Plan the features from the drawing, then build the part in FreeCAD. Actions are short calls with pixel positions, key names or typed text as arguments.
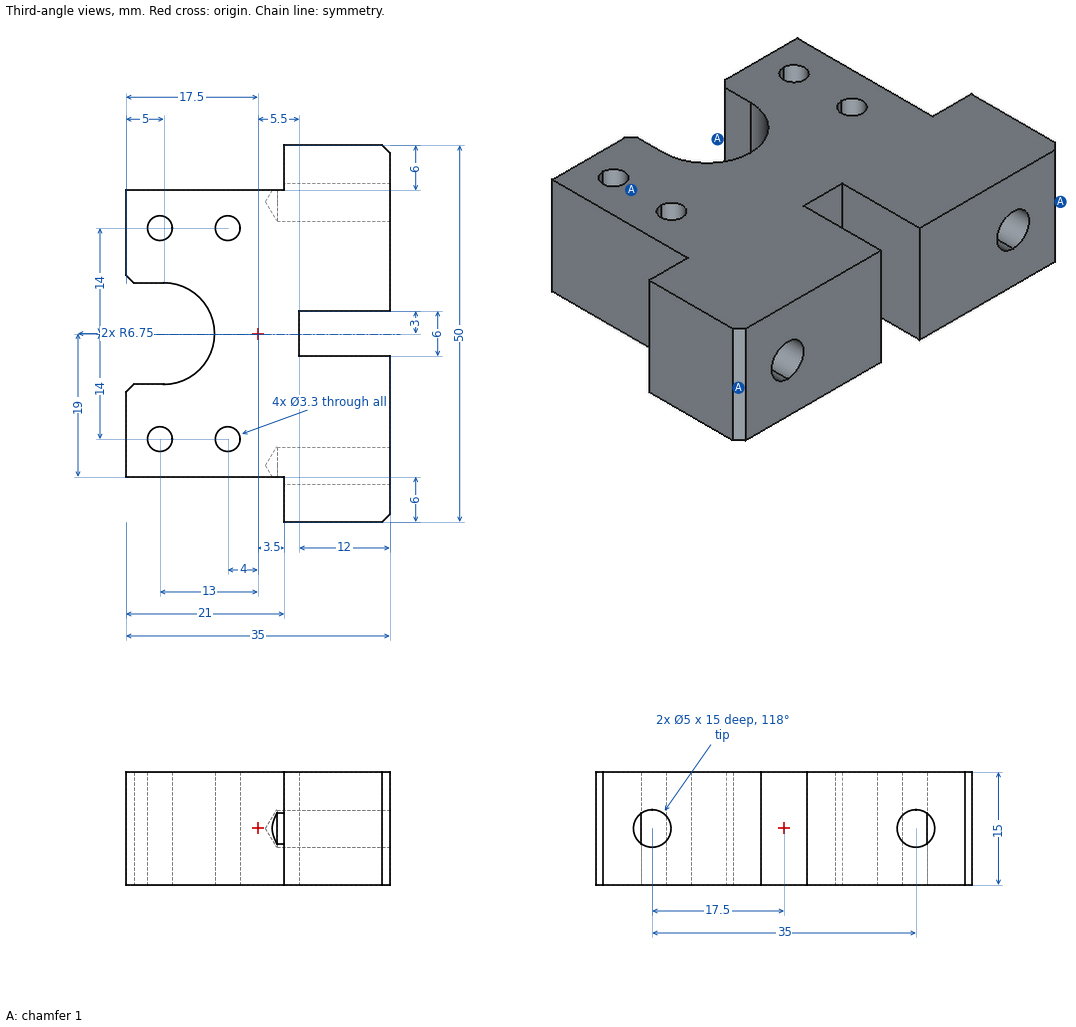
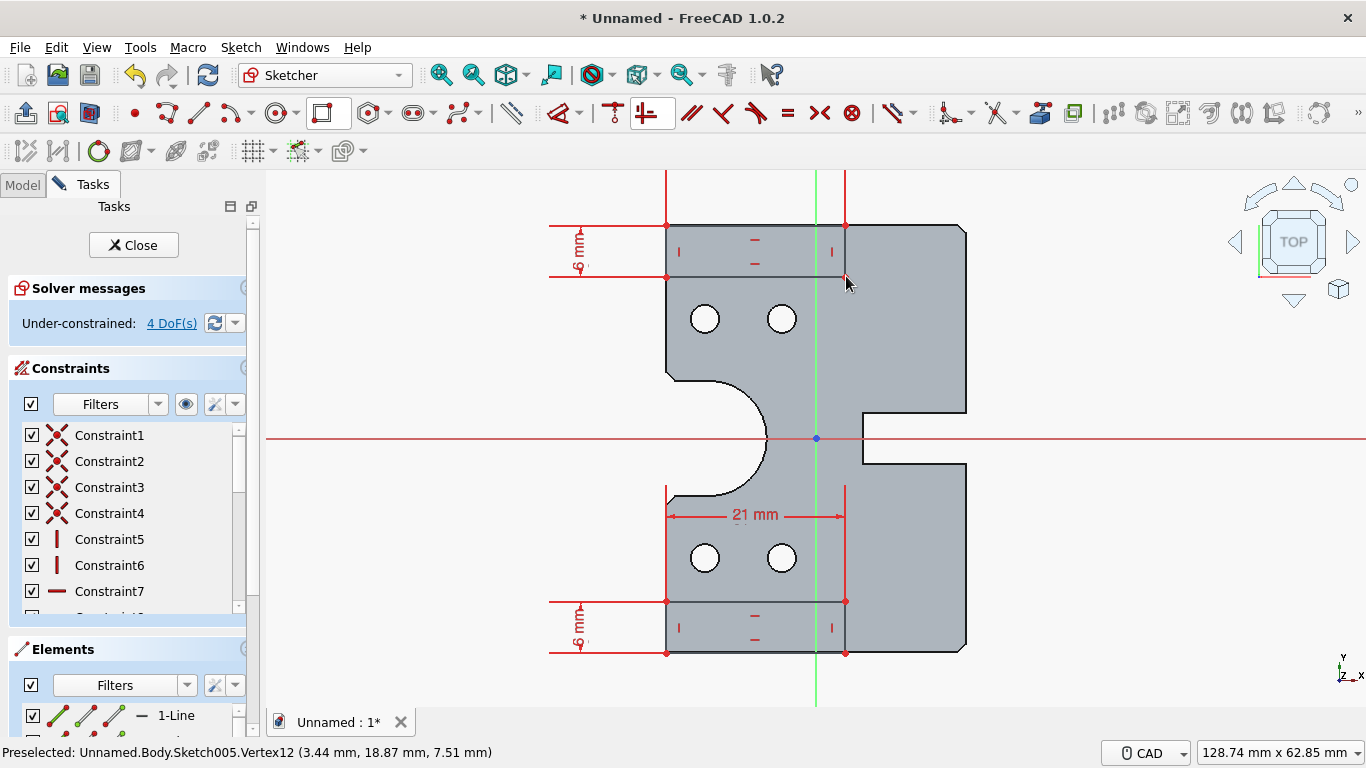
click(666, 653)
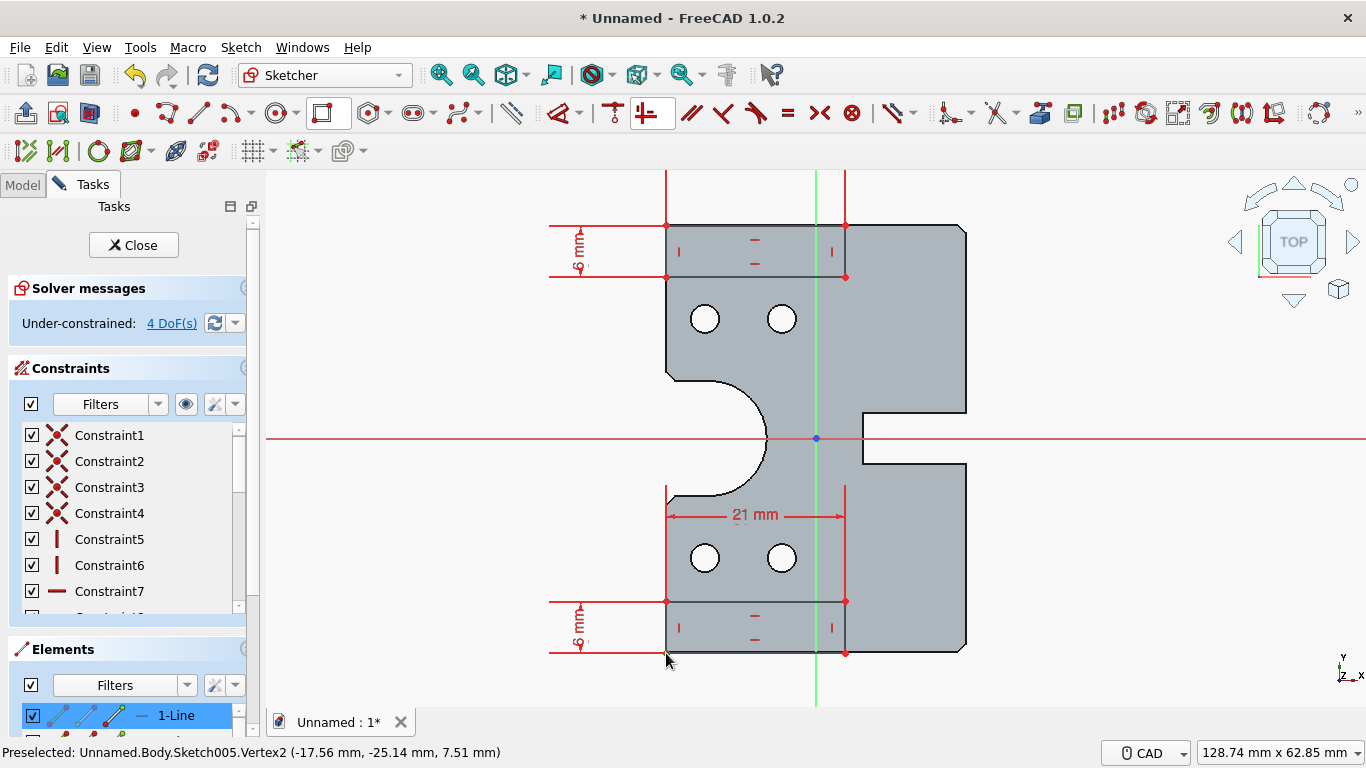
click(666, 226)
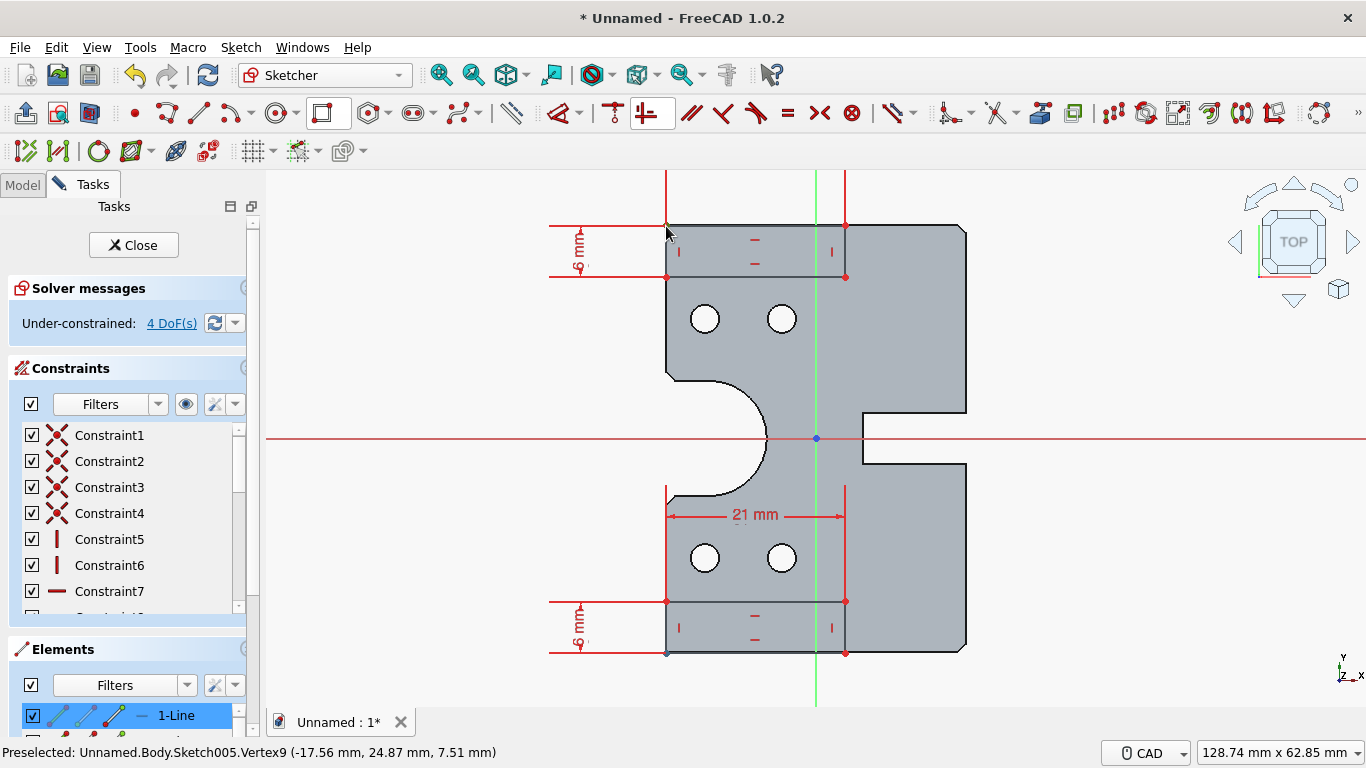
click(359, 438)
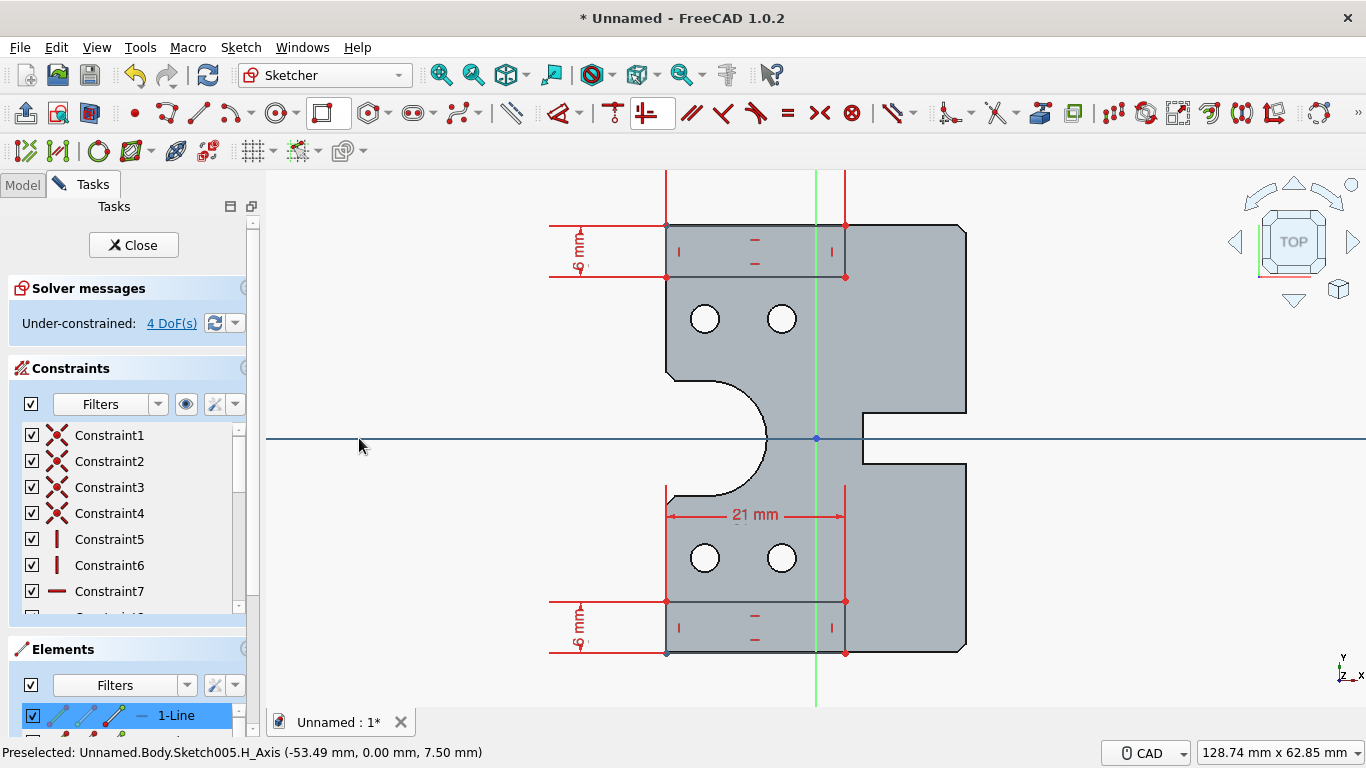
click(820, 114)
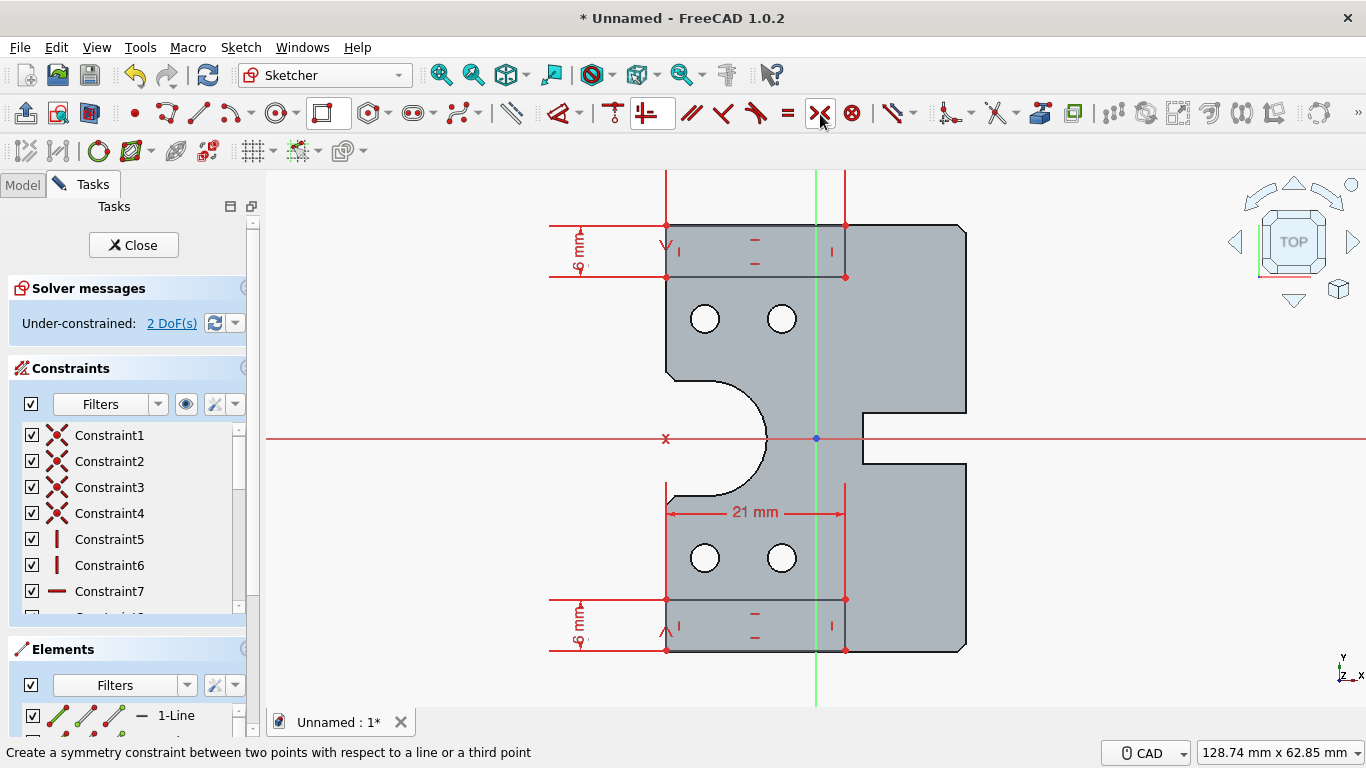
click(558, 114)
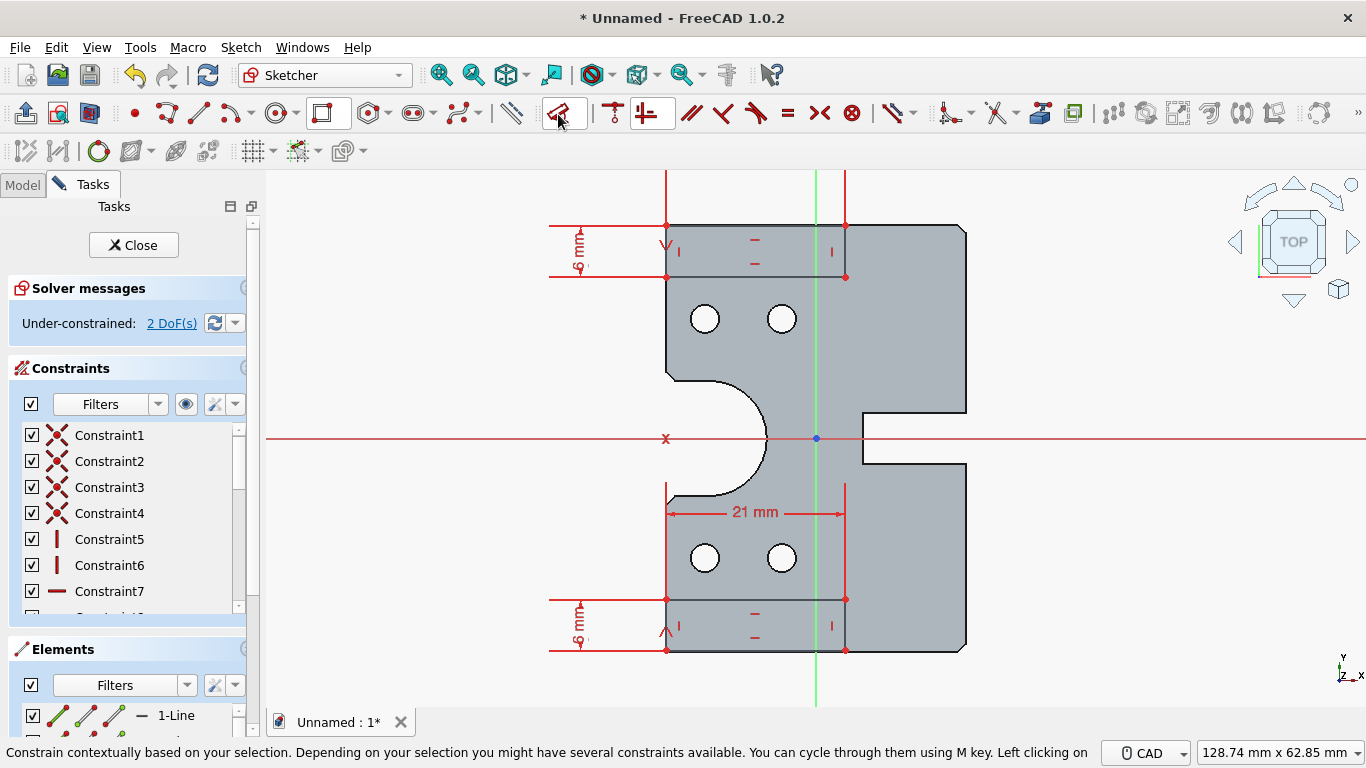
click(666, 600)
click(632, 519)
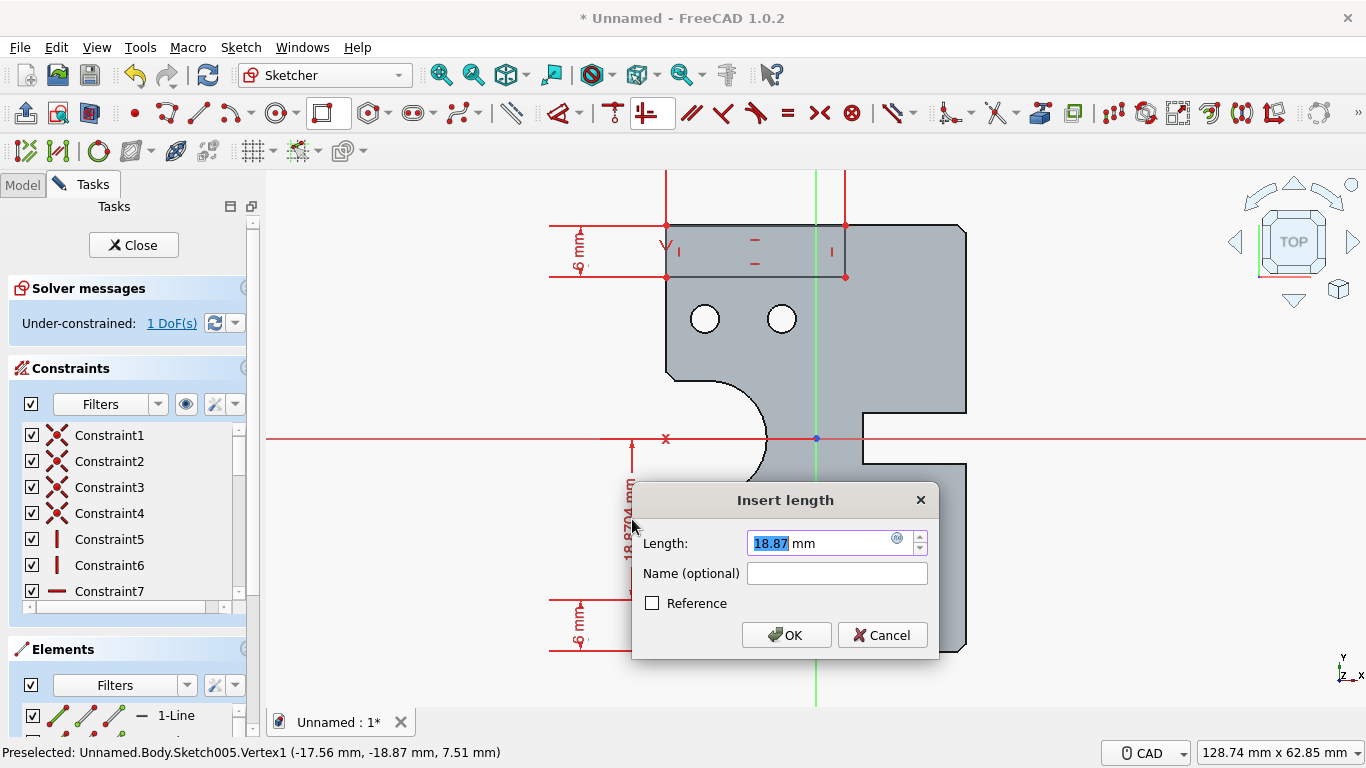
text(19)
key(Return)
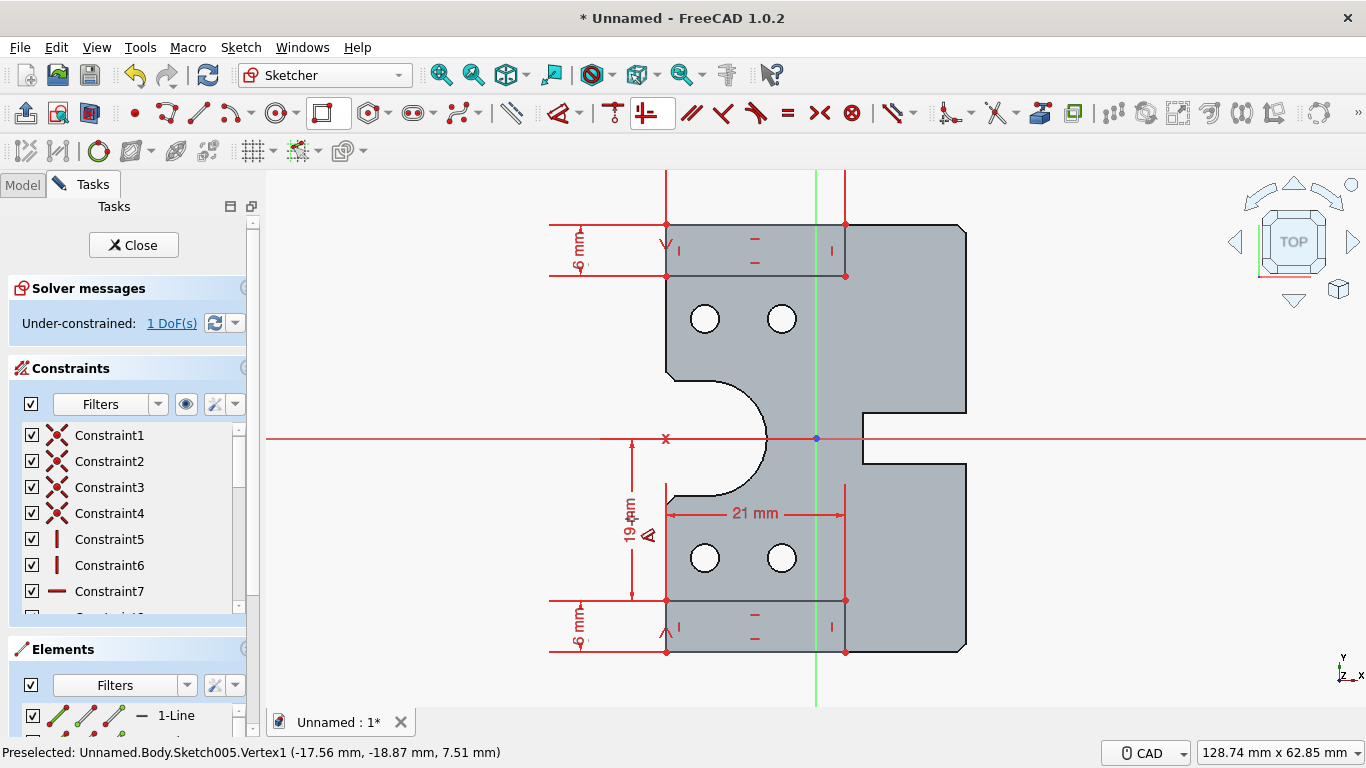
scroll(845, 652, up, 2)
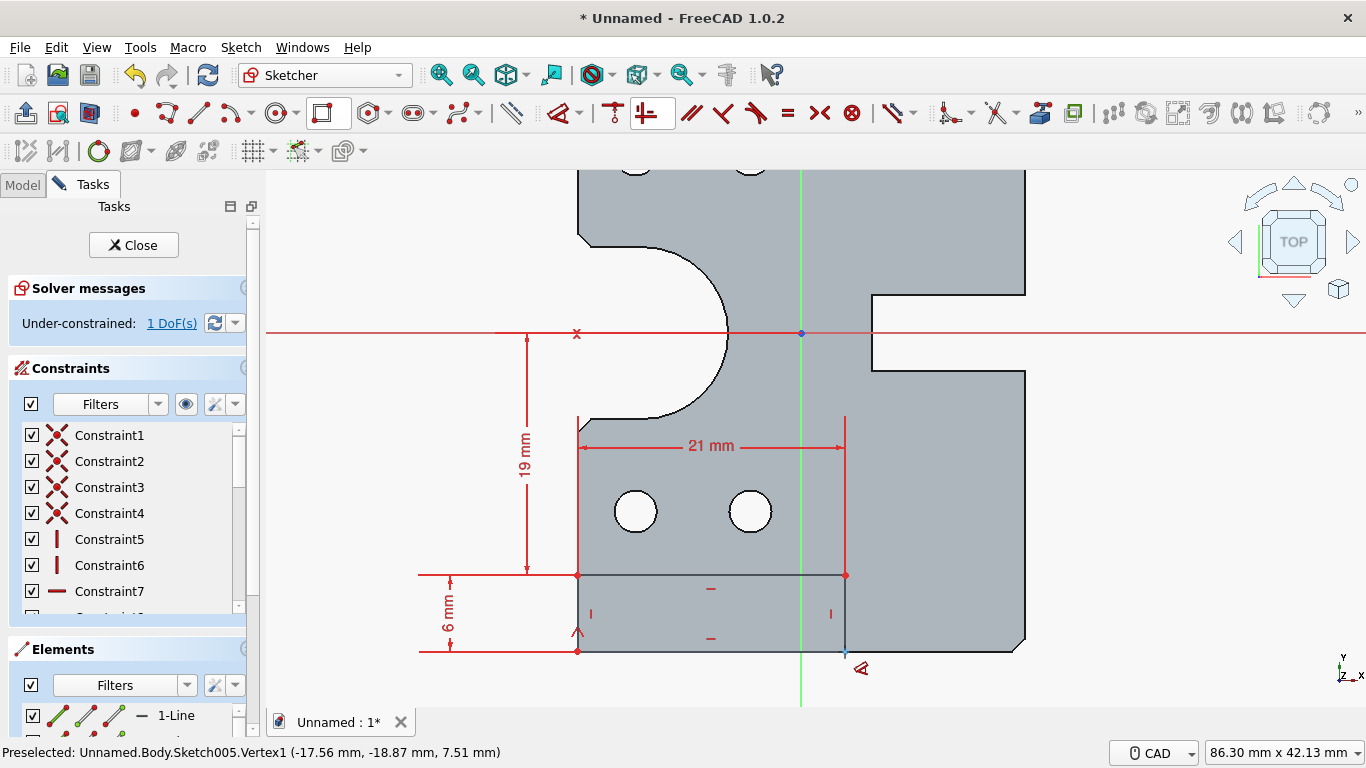
click(845, 652)
click(823, 299)